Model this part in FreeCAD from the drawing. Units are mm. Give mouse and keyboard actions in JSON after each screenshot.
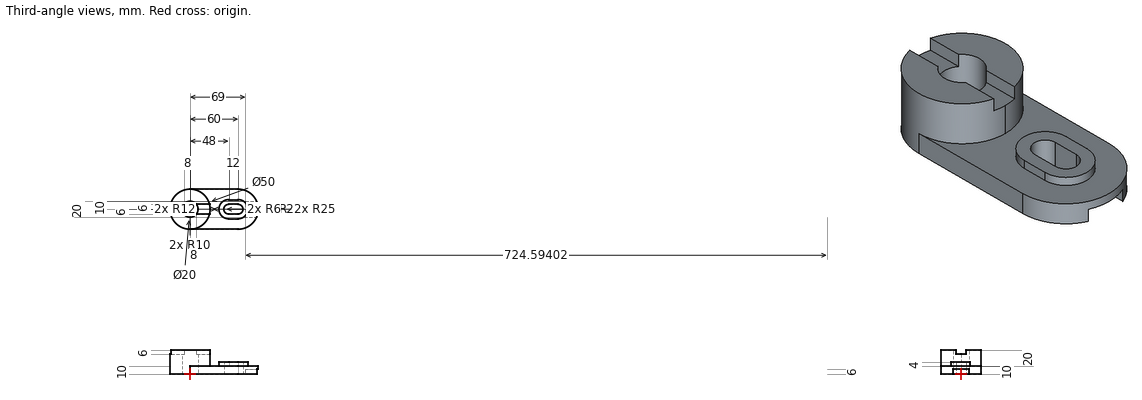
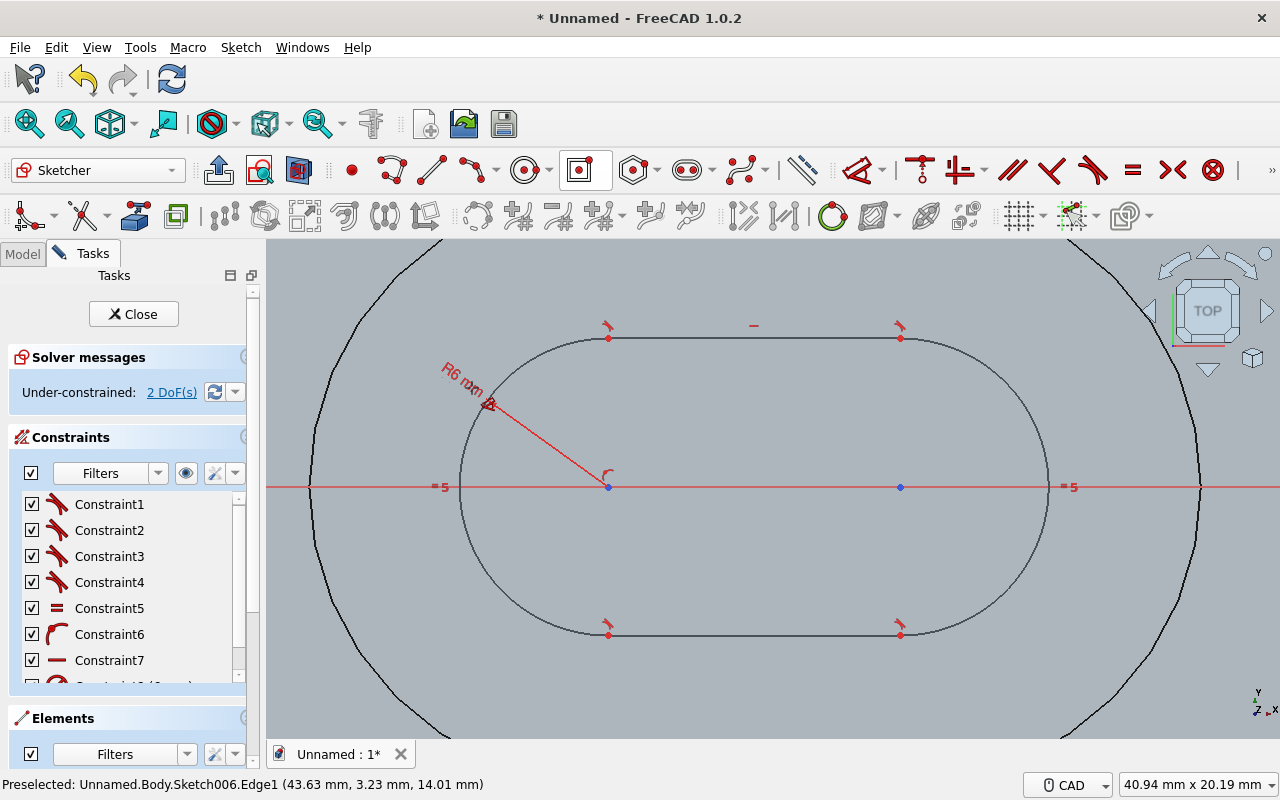
{"action": "left_click", "coordinate": [696, 338]}
{"action": "left_click", "coordinate": [754, 304]}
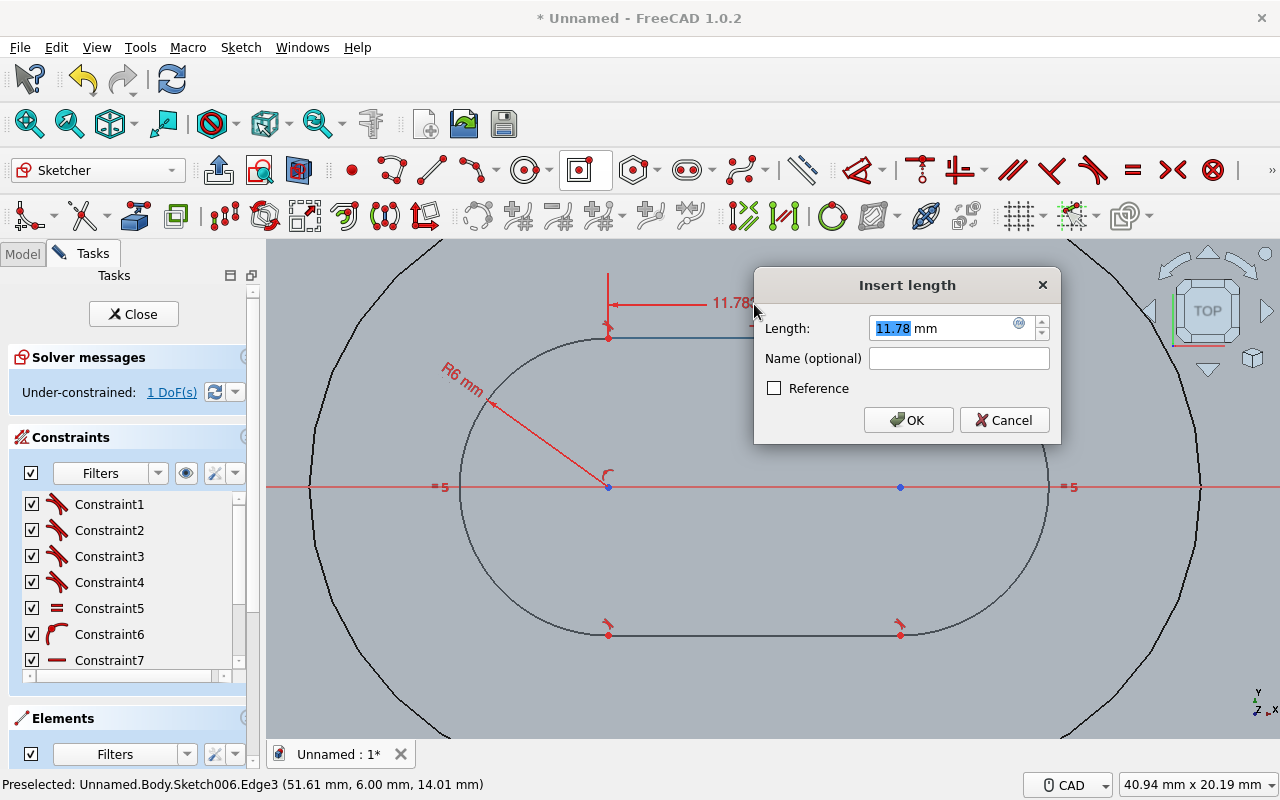
{"action": "type", "text": "12"}
{"action": "key", "text": "Return"}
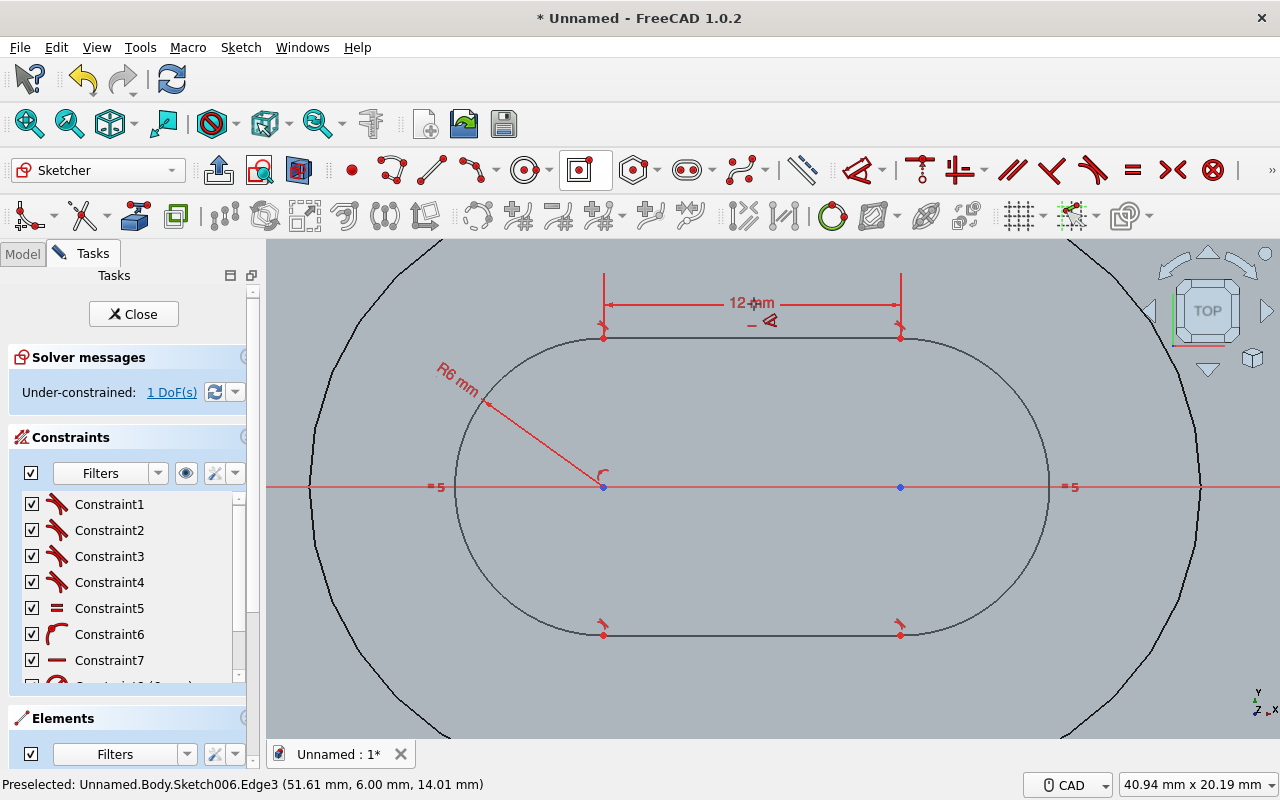
{"action": "left_click", "coordinate": [604, 338]}
{"action": "left_click", "coordinate": [449, 304]}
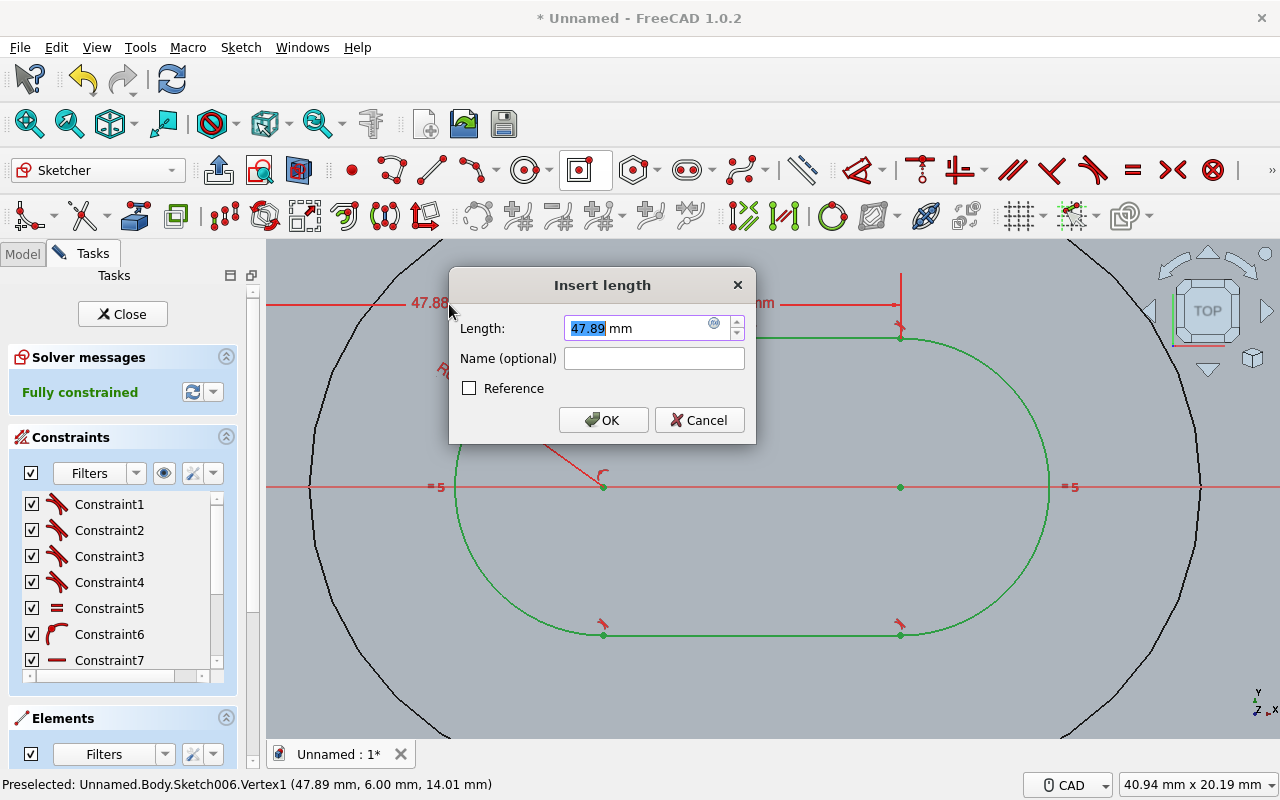
{"action": "type", "text": "48"}
{"action": "key", "text": "Return"}
{"action": "key", "text": "Escape"}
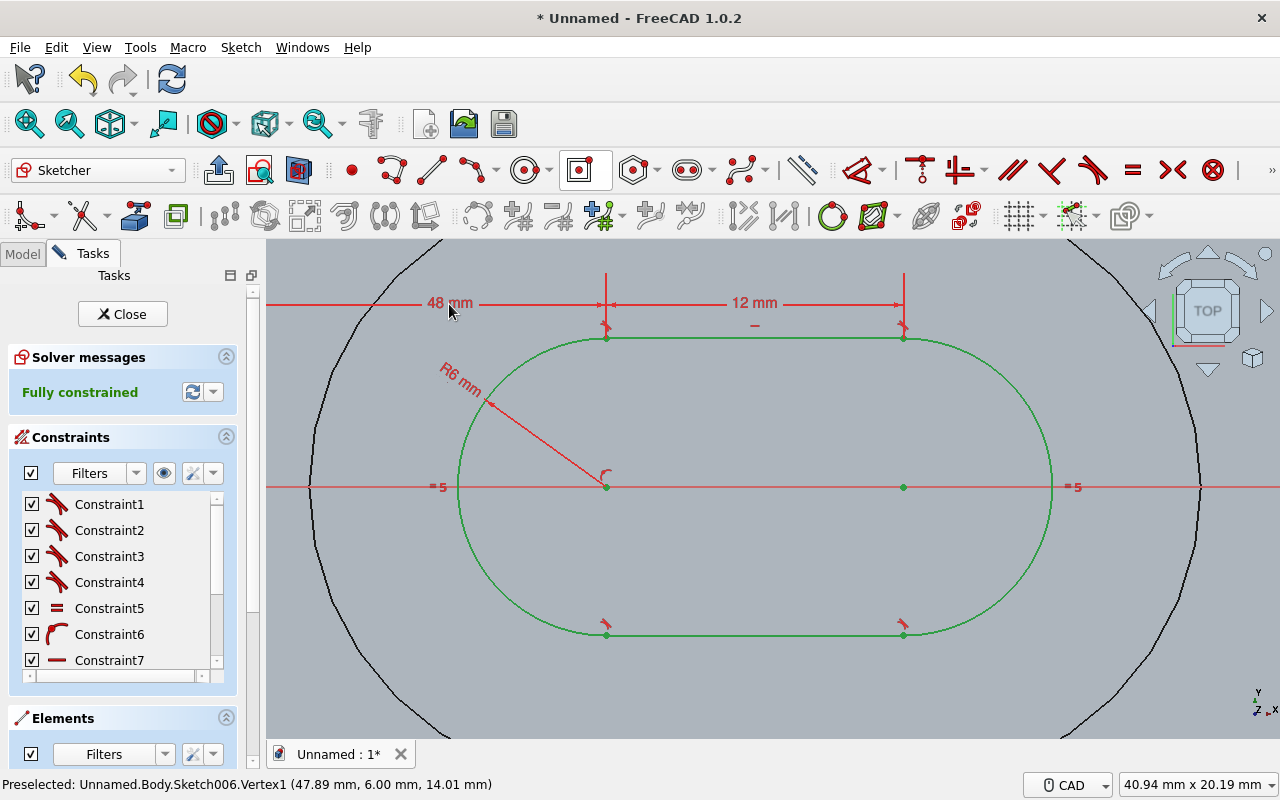
{"action": "left_click", "coordinate": [123, 314]}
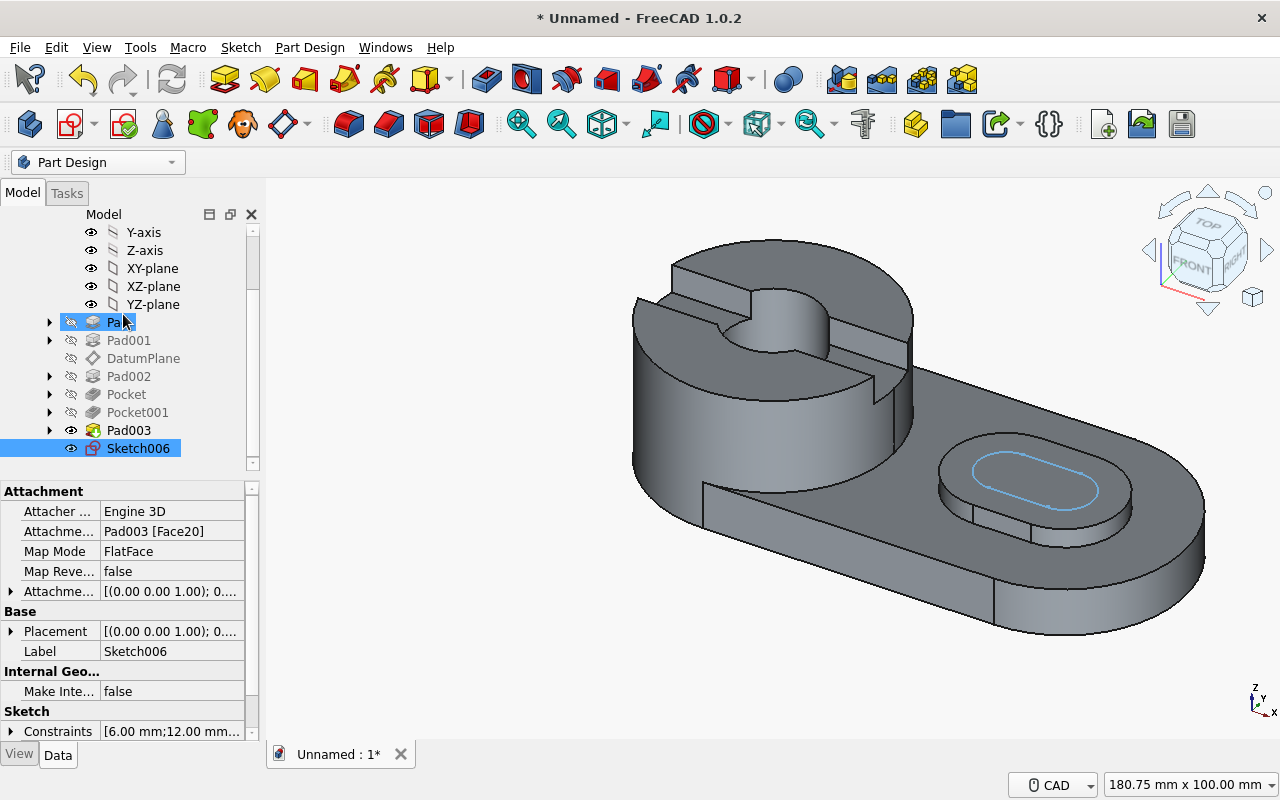
{"action": "left_click", "coordinate": [488, 80]}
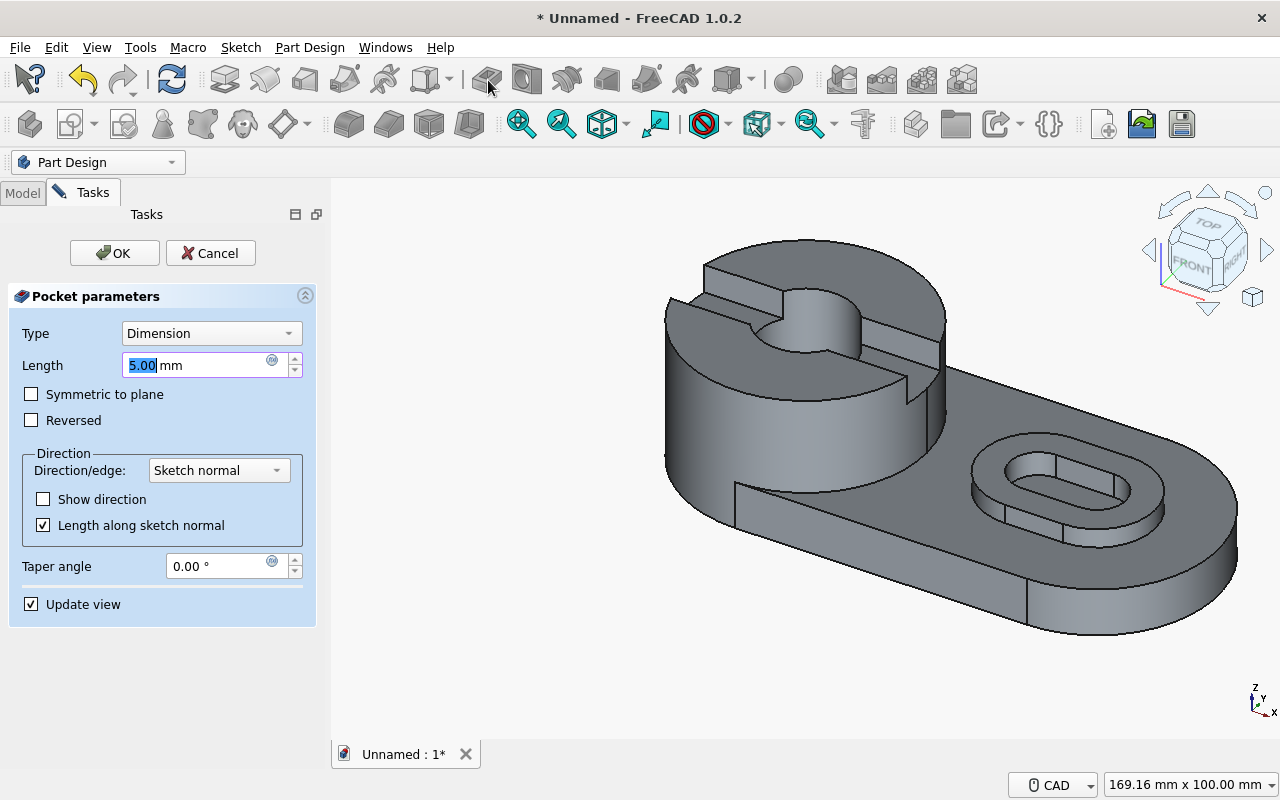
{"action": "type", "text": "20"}
{"action": "key", "text": "Tab"}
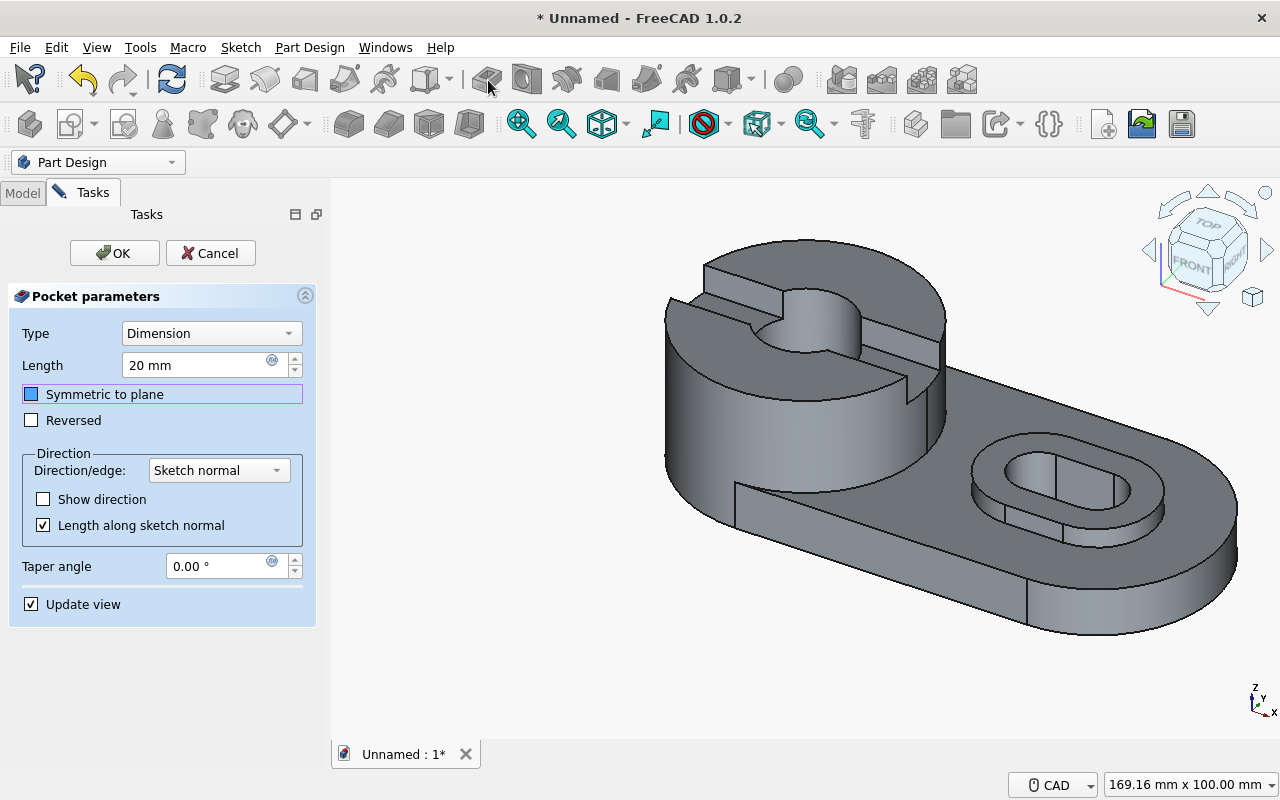
{"action": "left_click", "coordinate": [115, 253]}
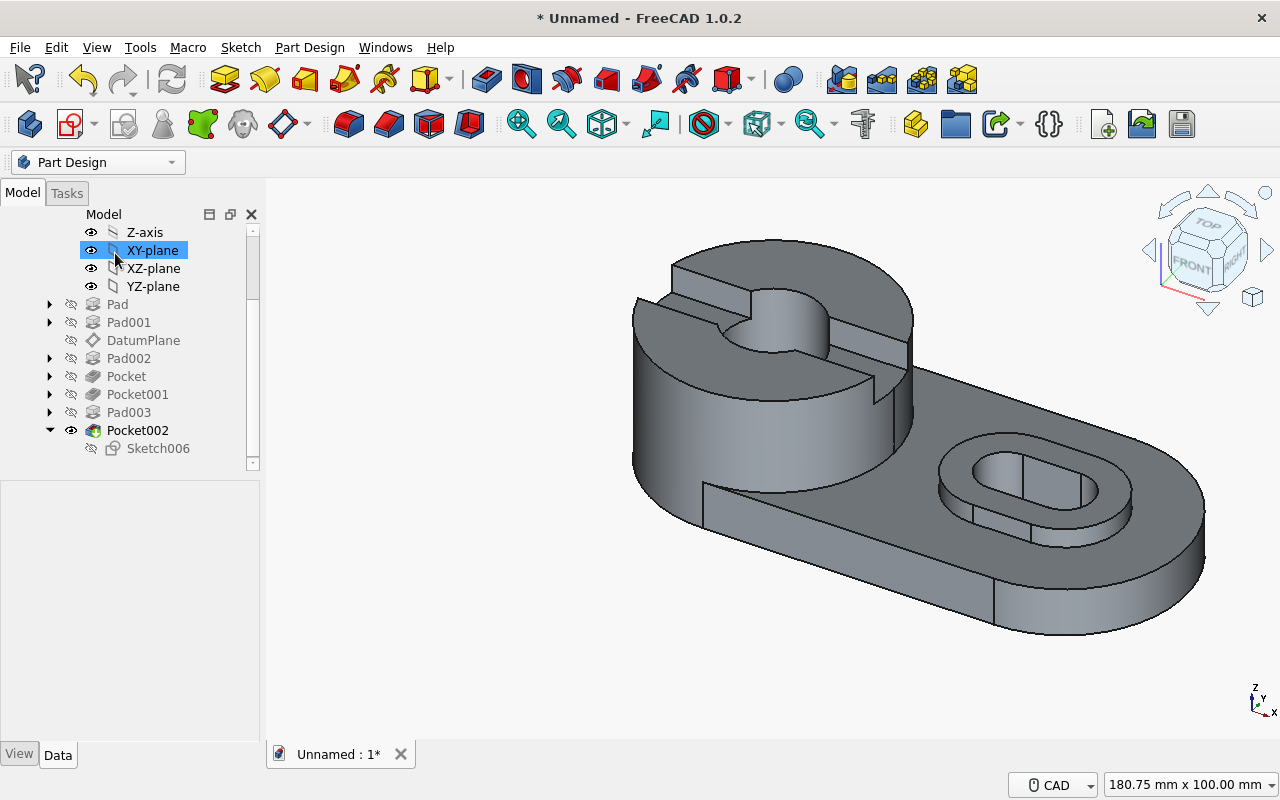
{"action": "left_click", "coordinate": [70, 124]}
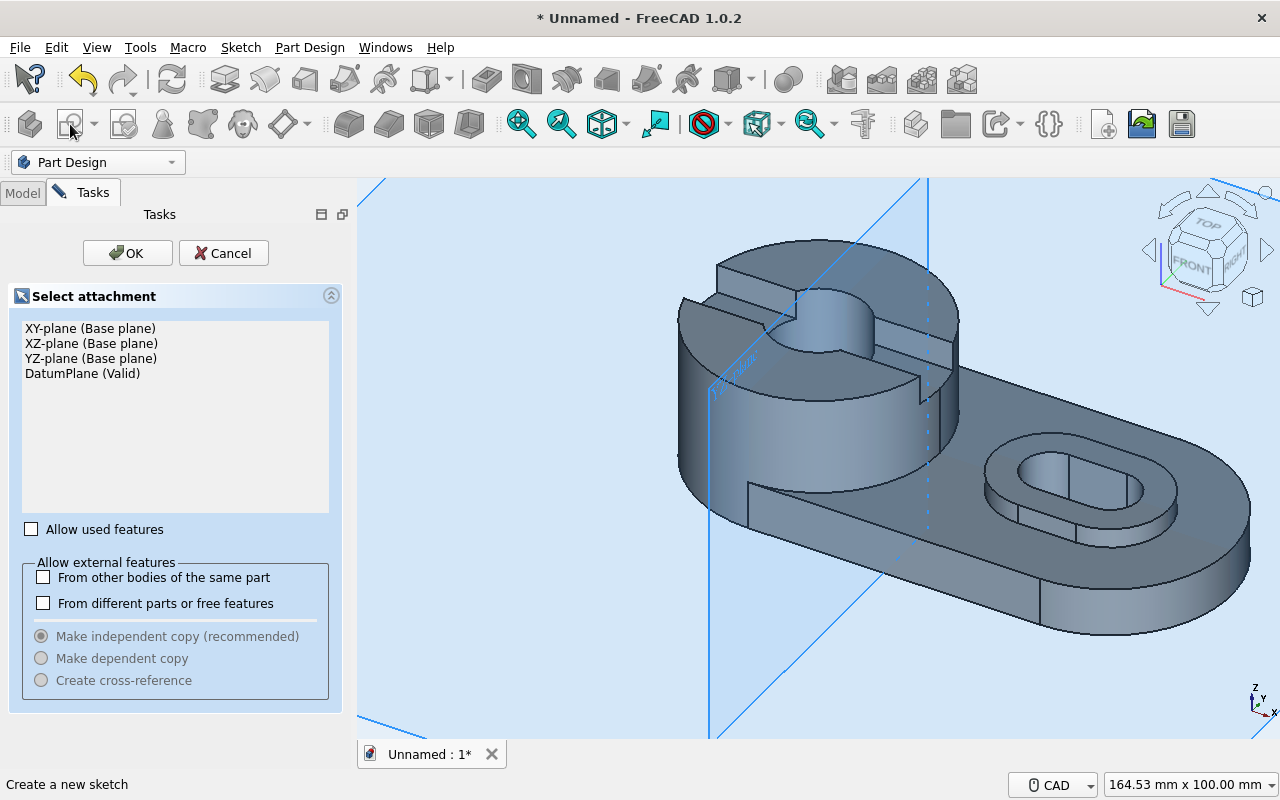
{"action": "left_click", "coordinate": [82, 328]}